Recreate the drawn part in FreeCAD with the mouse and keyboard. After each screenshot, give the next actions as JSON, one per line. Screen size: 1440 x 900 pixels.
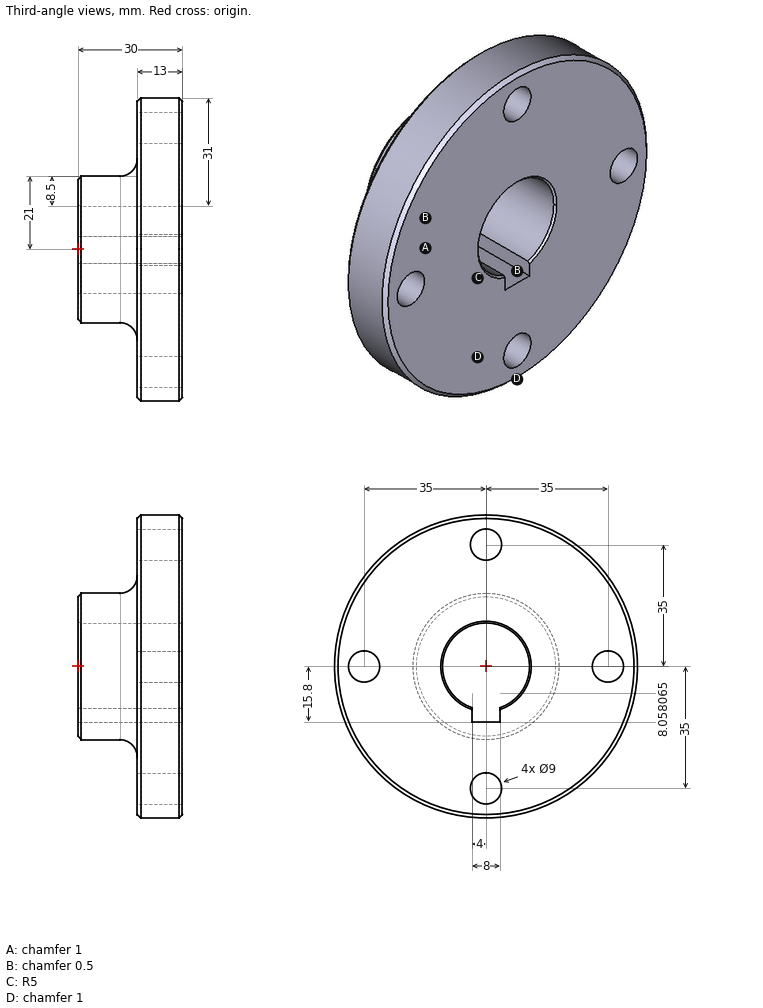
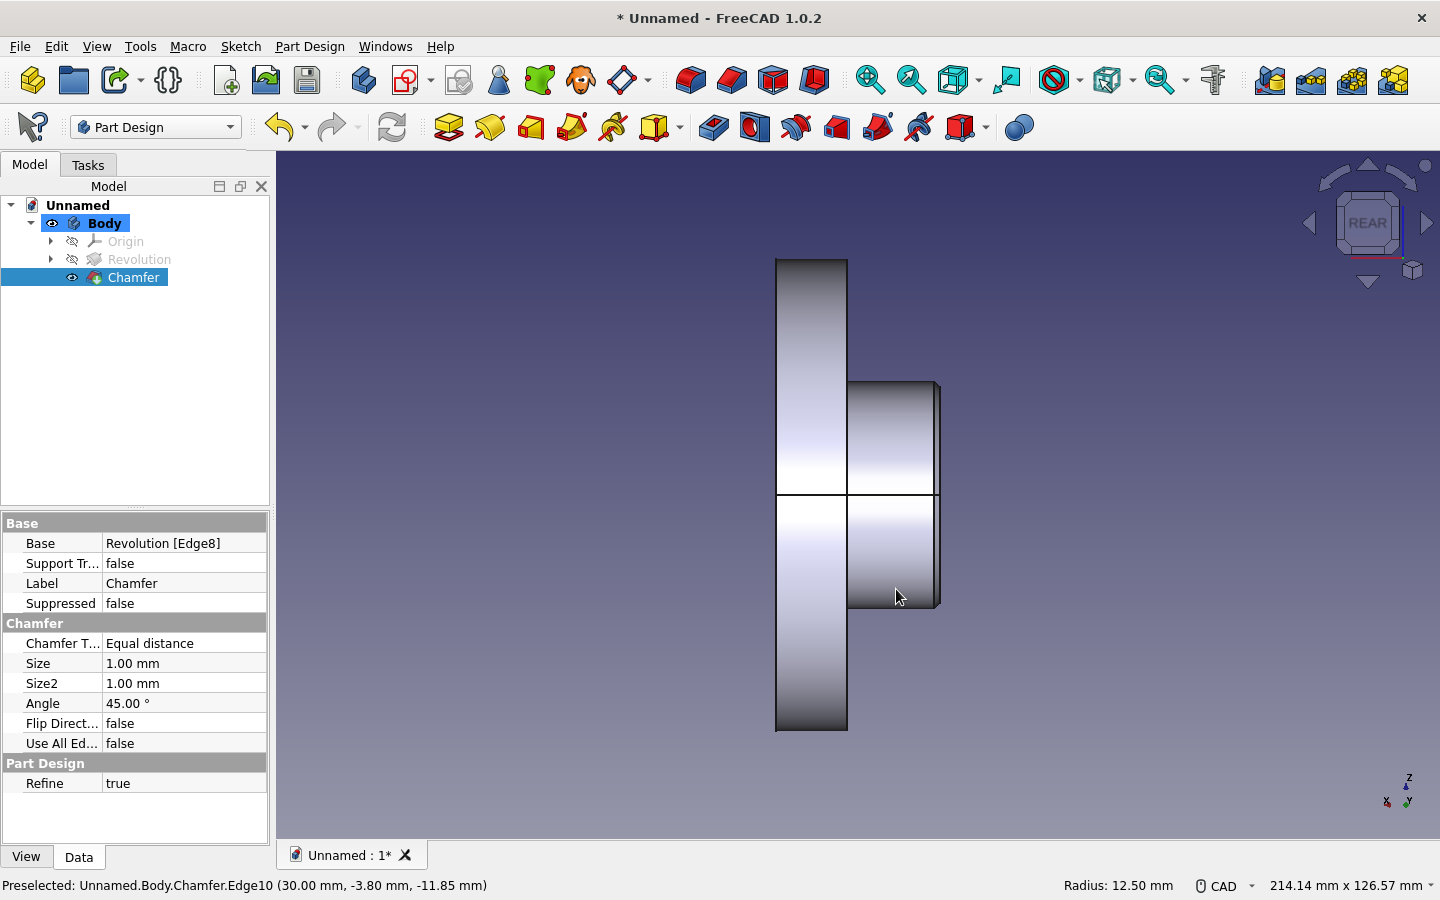
{"action": "key", "text": "6"}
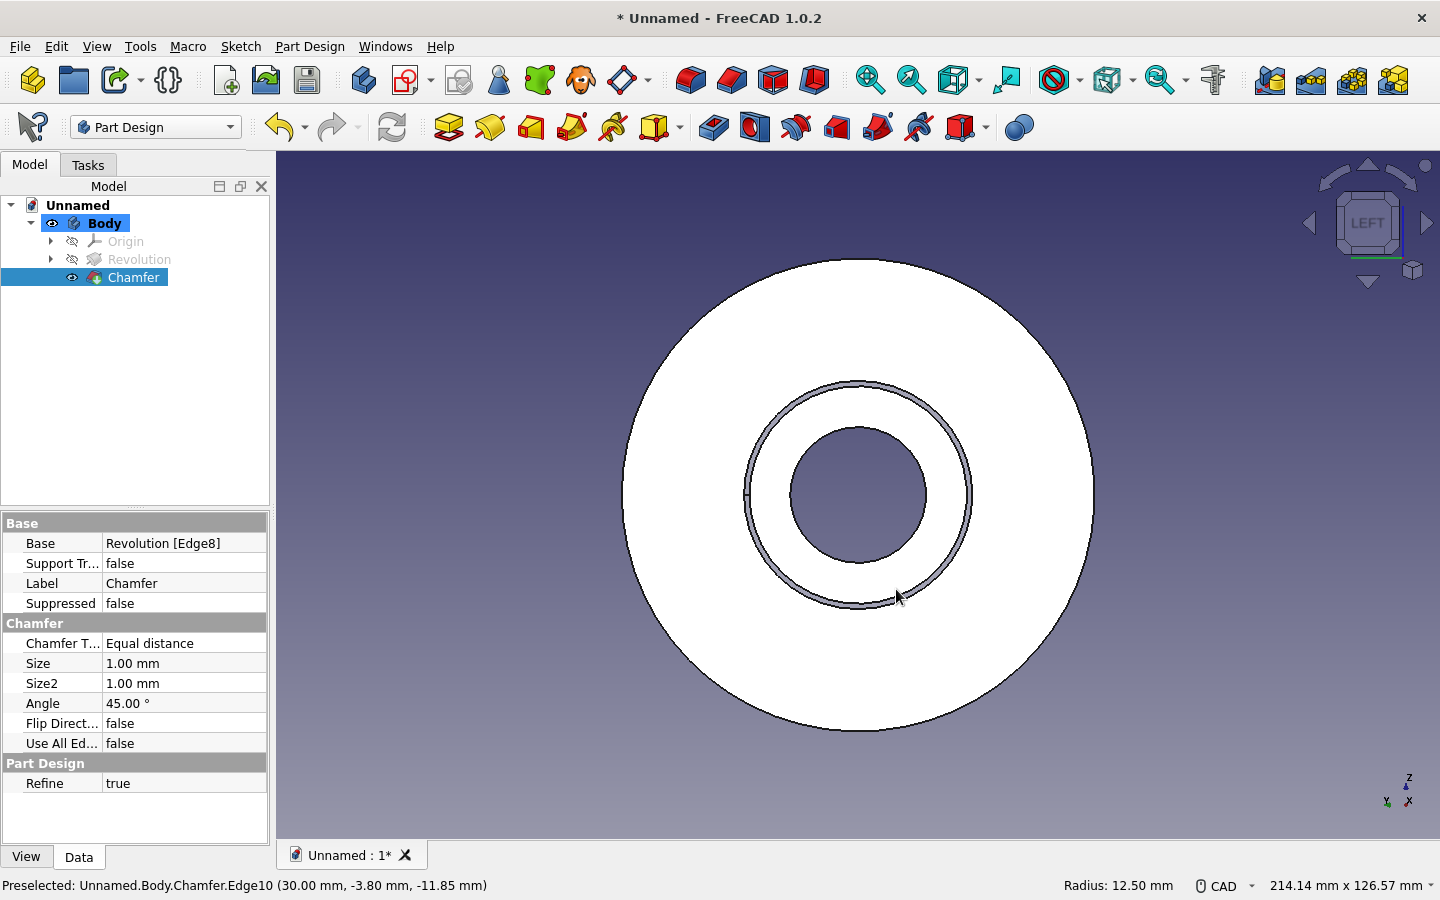
{"action": "left_click", "coordinate": [913, 454], "text": "ctrl"}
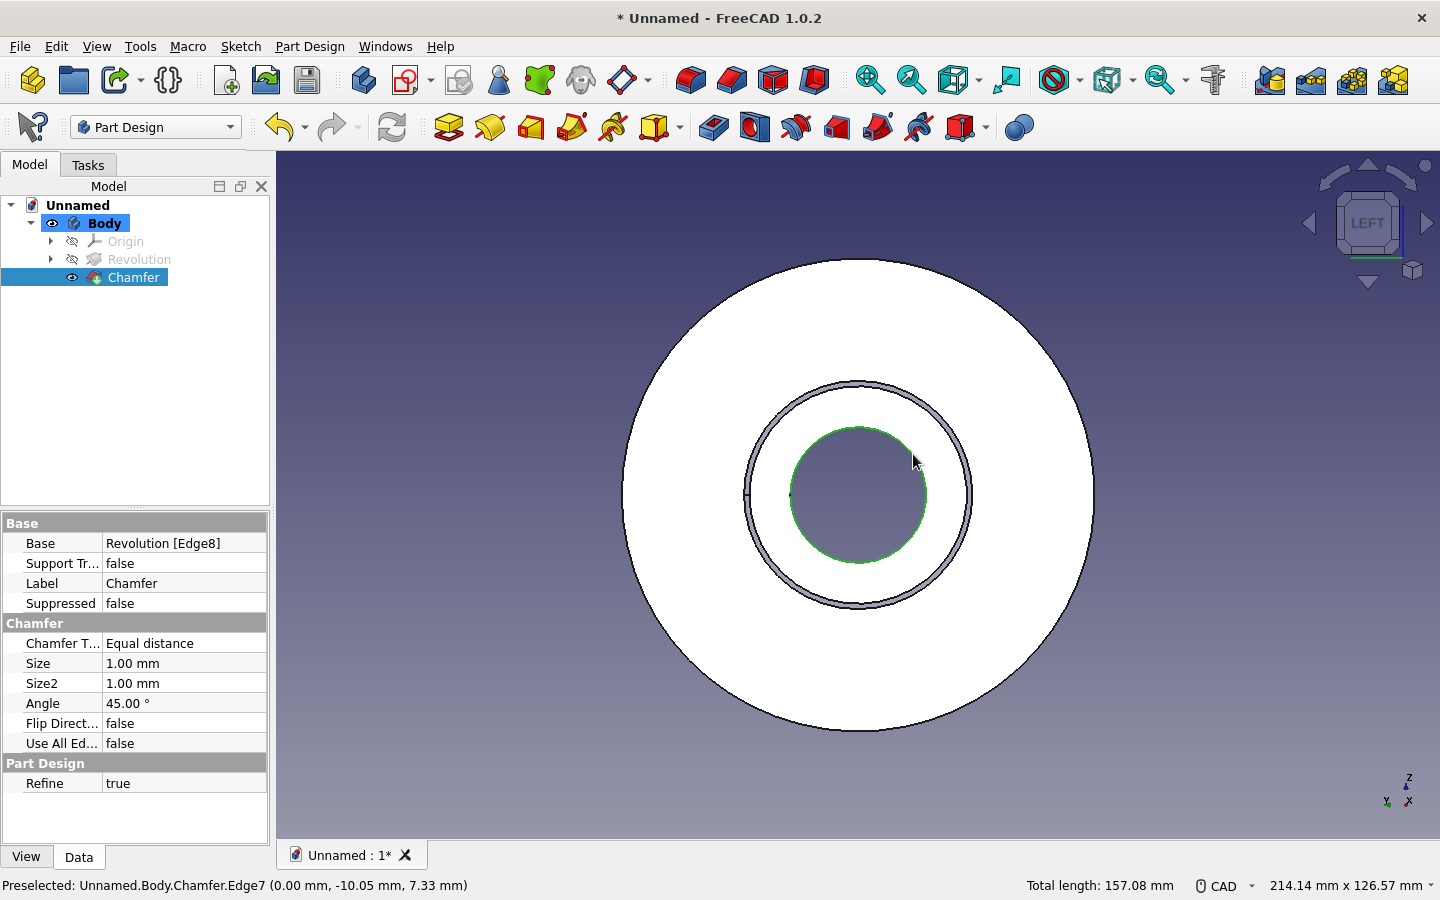
{"action": "left_click", "coordinate": [732, 80]}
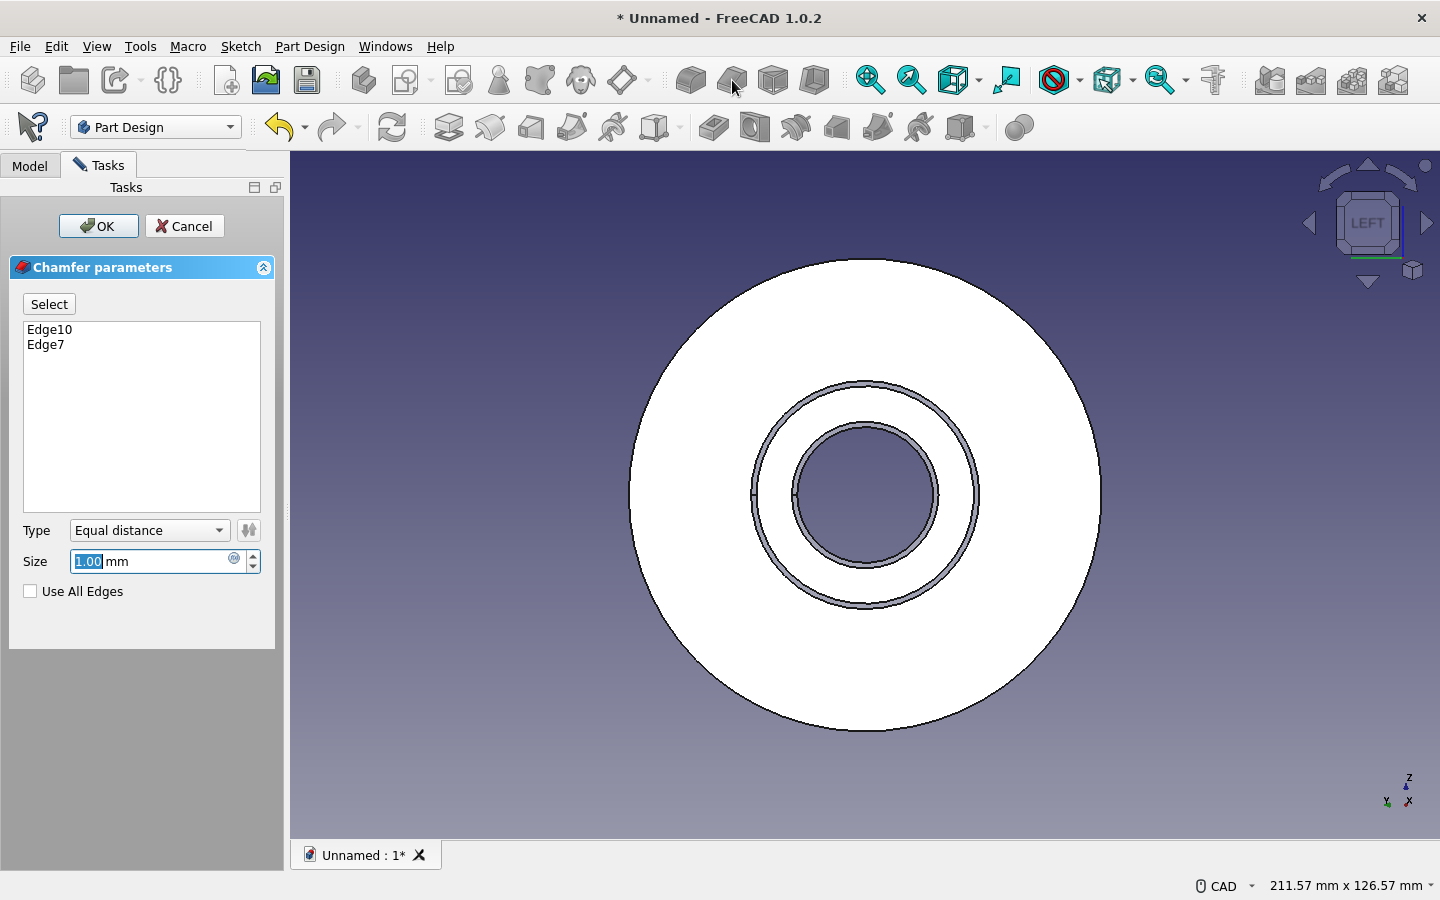
{"action": "type", "text": "0.5"}
{"action": "key", "text": "Tab"}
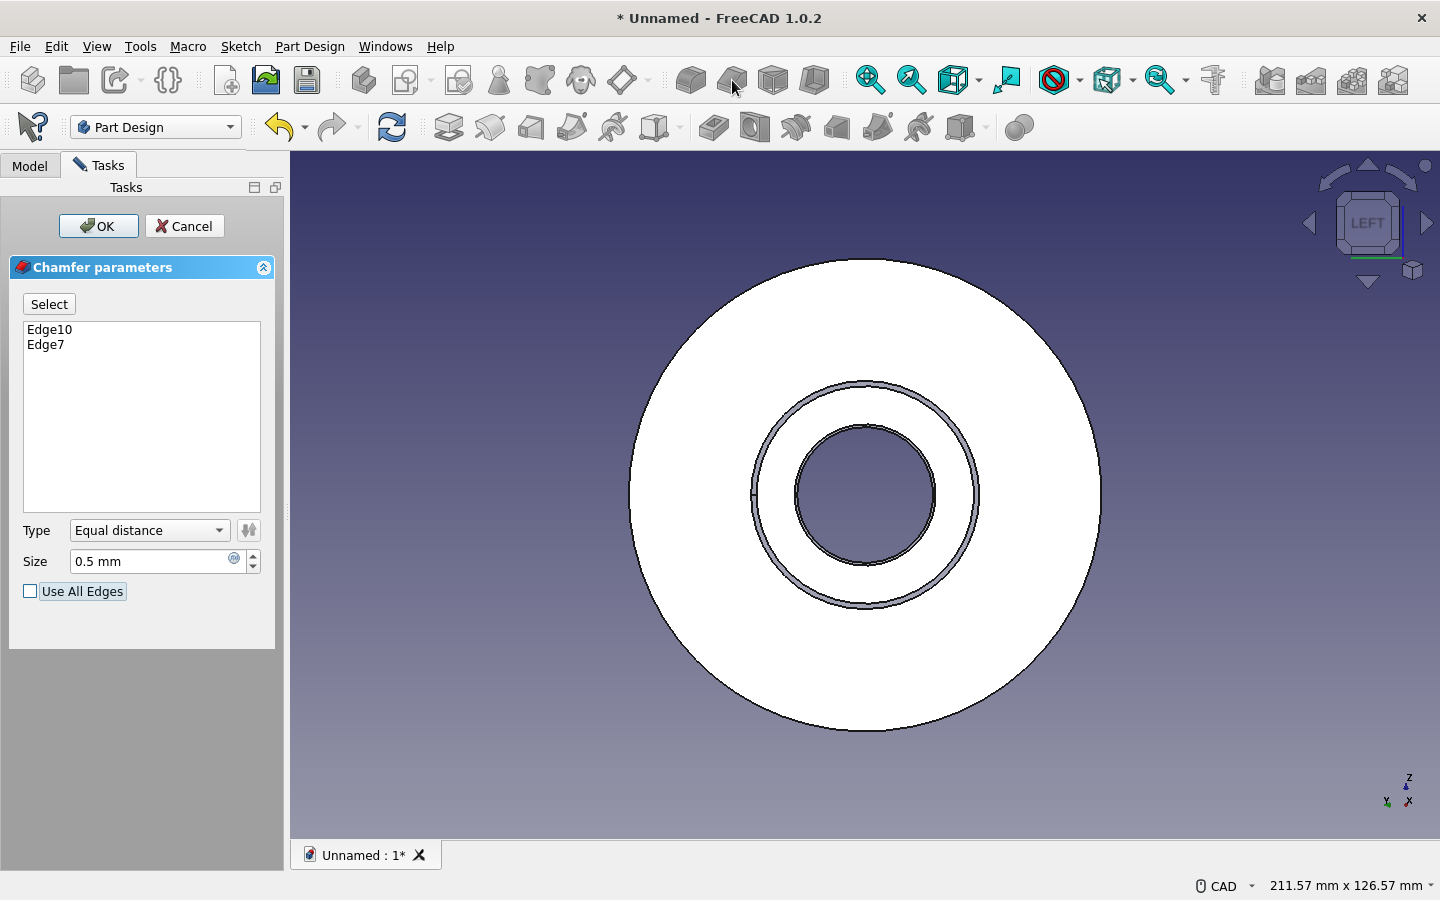
{"action": "left_click", "coordinate": [99, 226]}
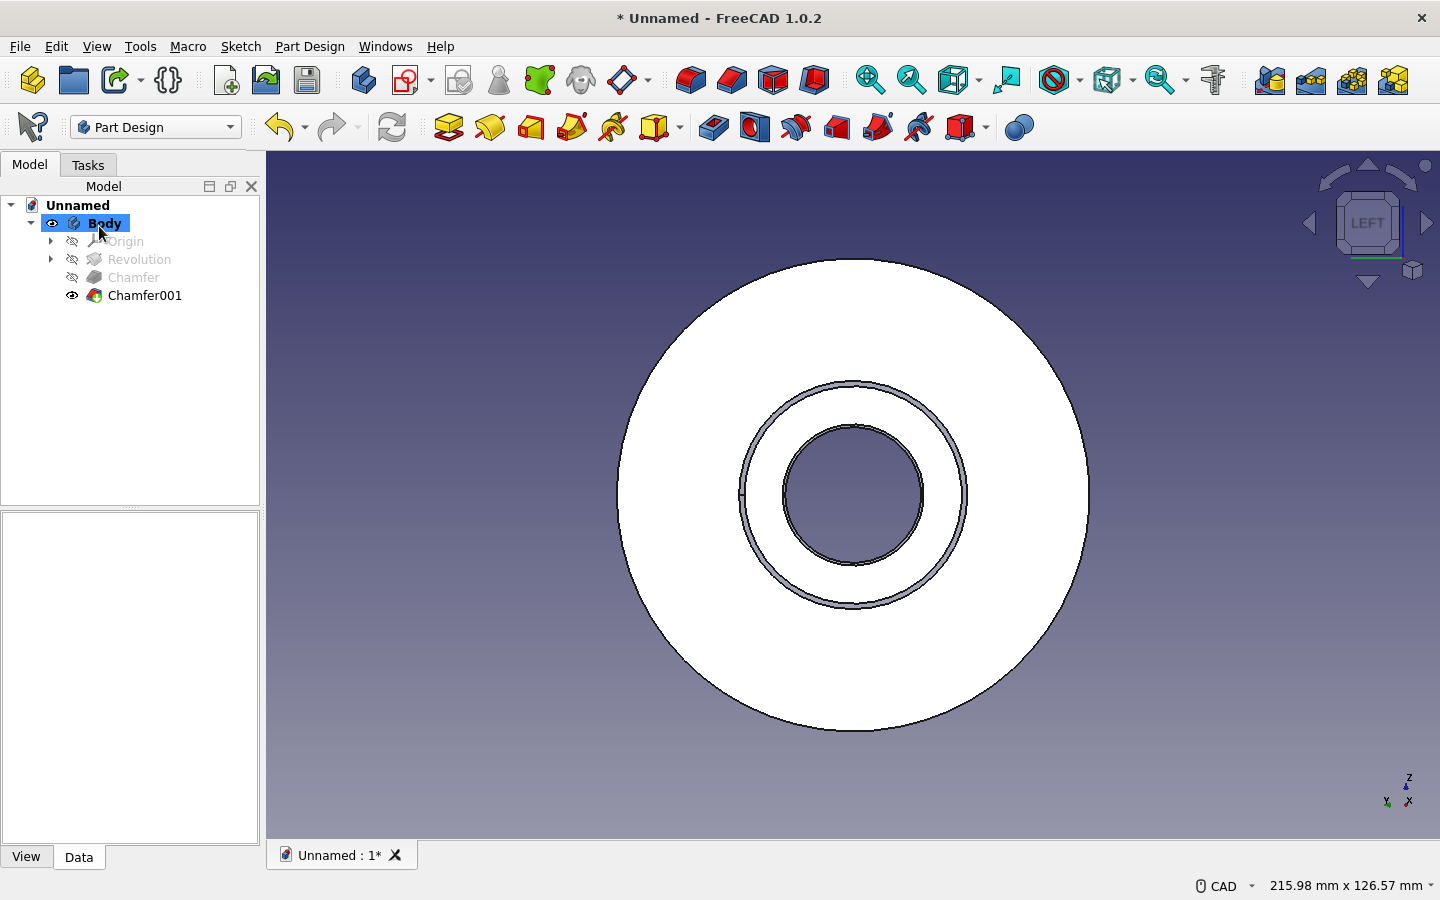
{"action": "key", "text": "0"}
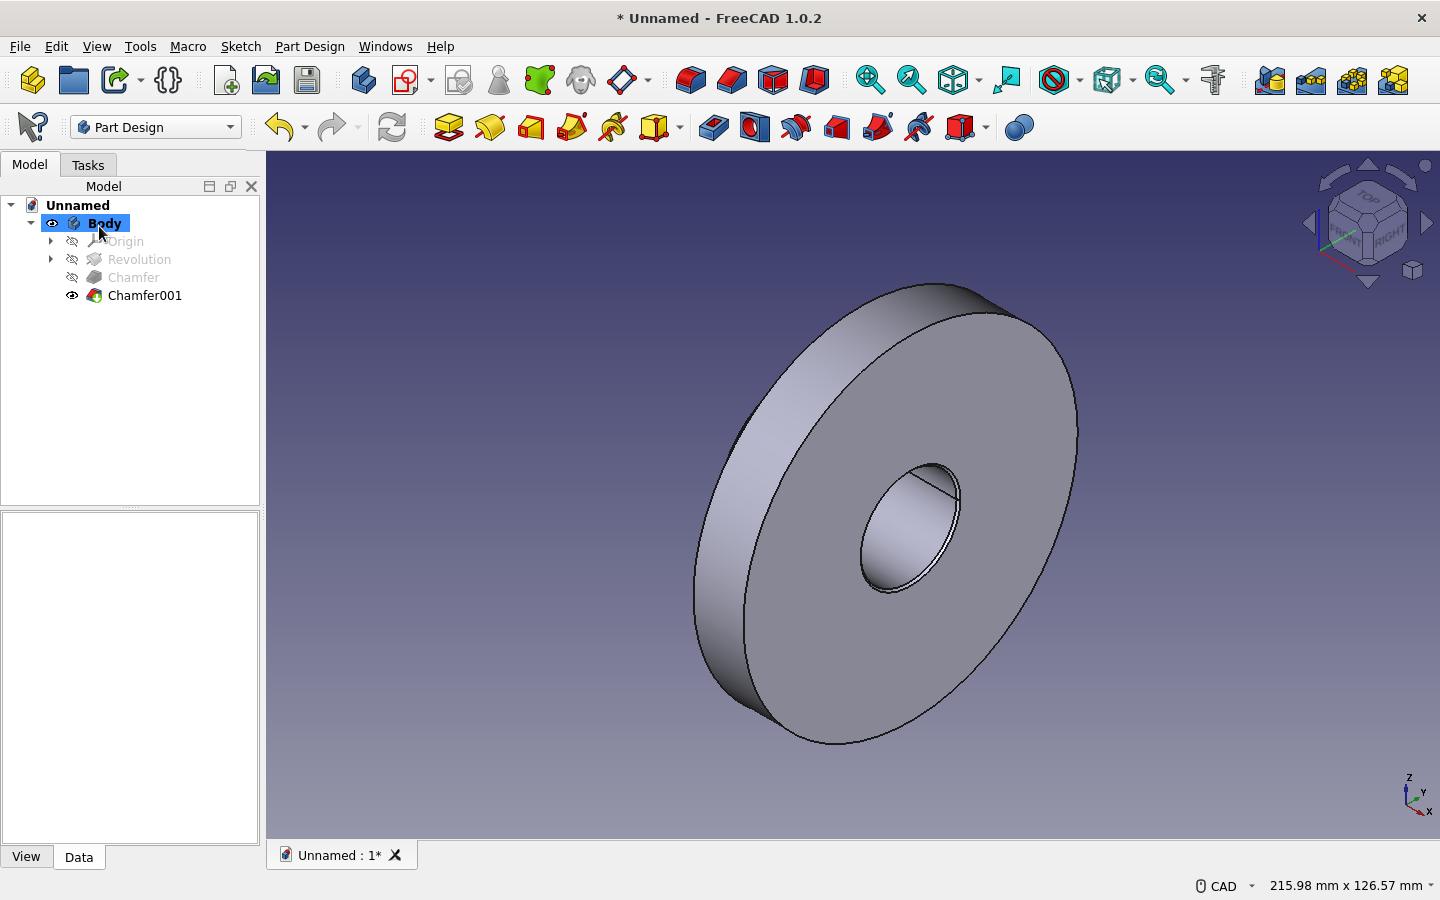
{"action": "key", "text": "2"}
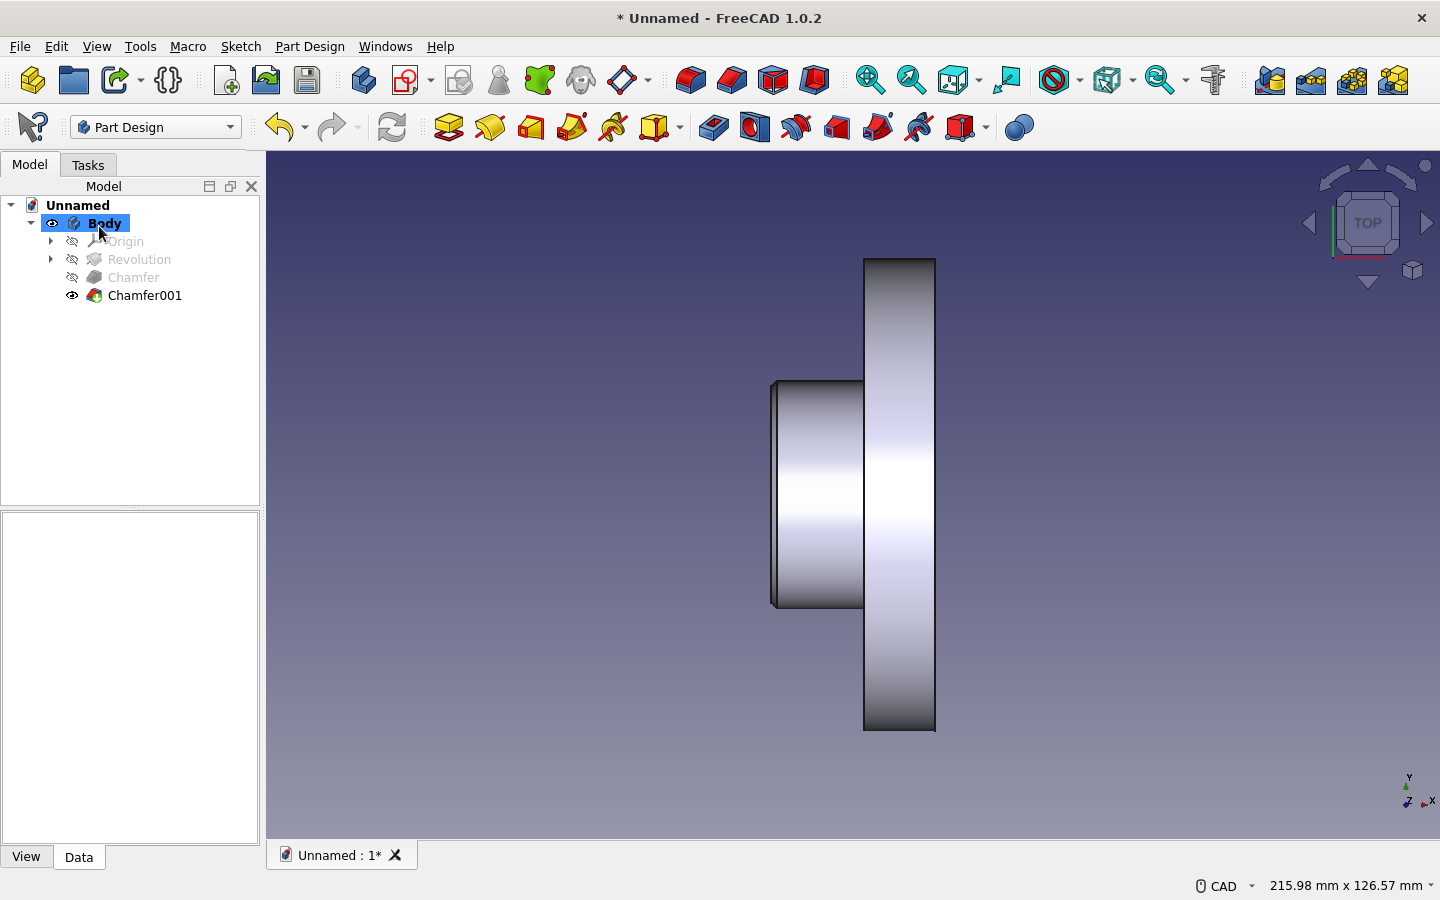
{"action": "key", "text": "1"}